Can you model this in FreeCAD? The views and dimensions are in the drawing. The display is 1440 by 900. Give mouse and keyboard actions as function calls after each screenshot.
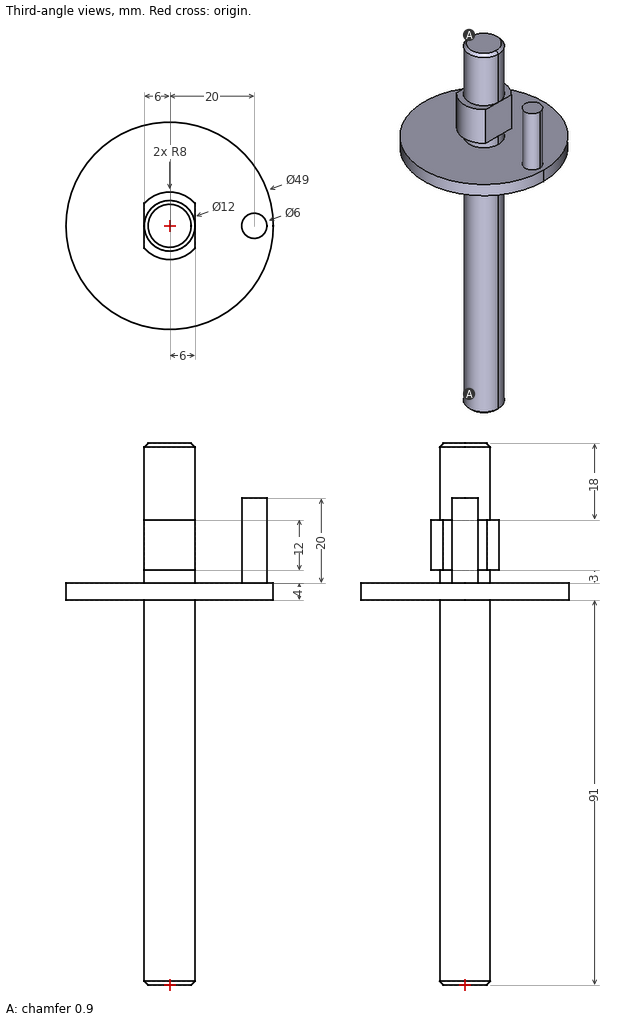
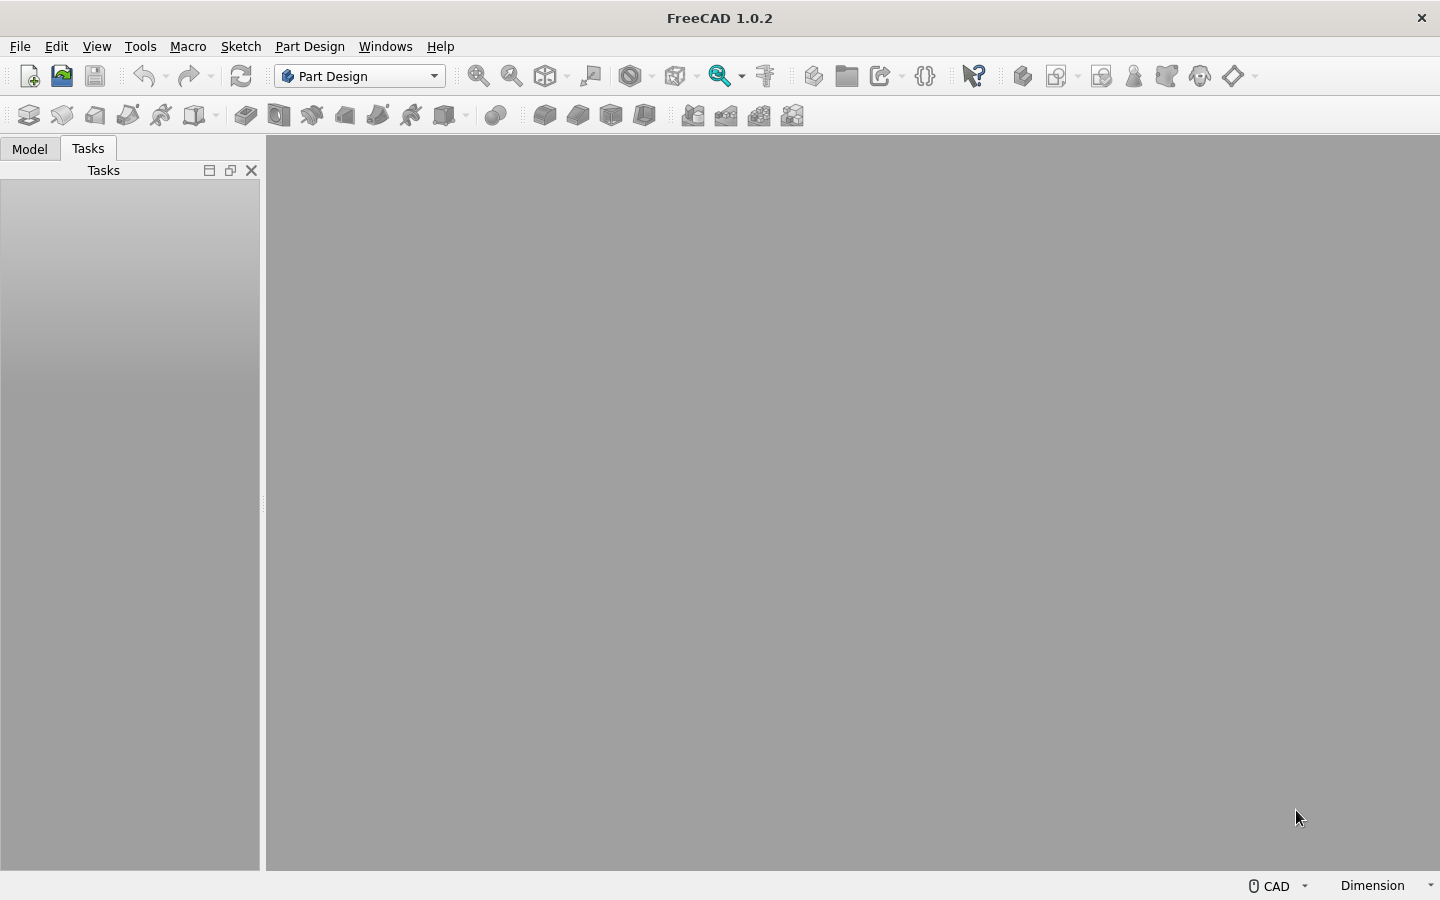
key(ctrl+n)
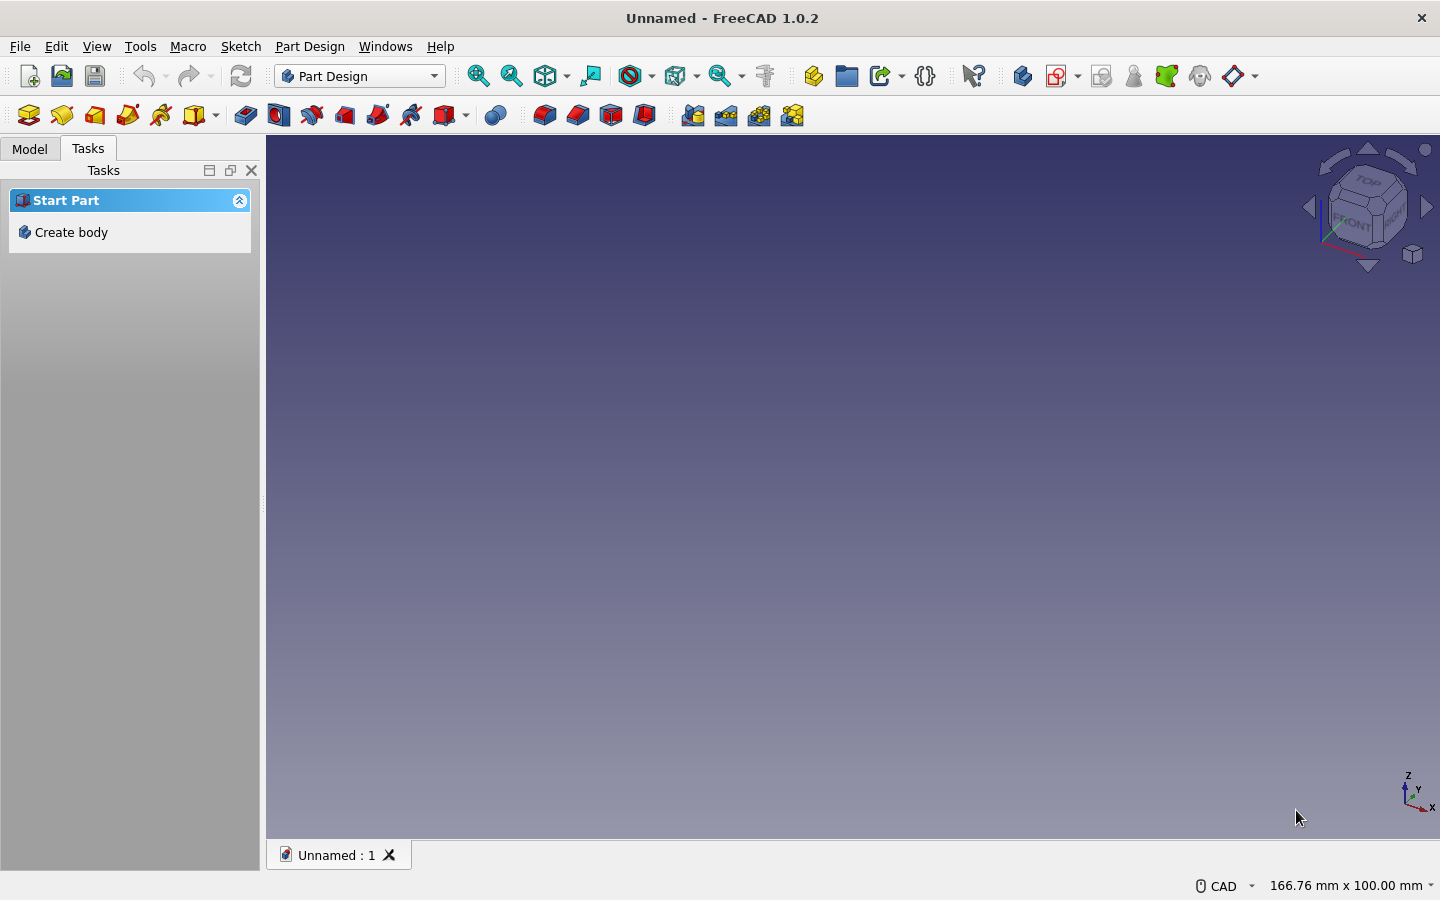
click(1056, 76)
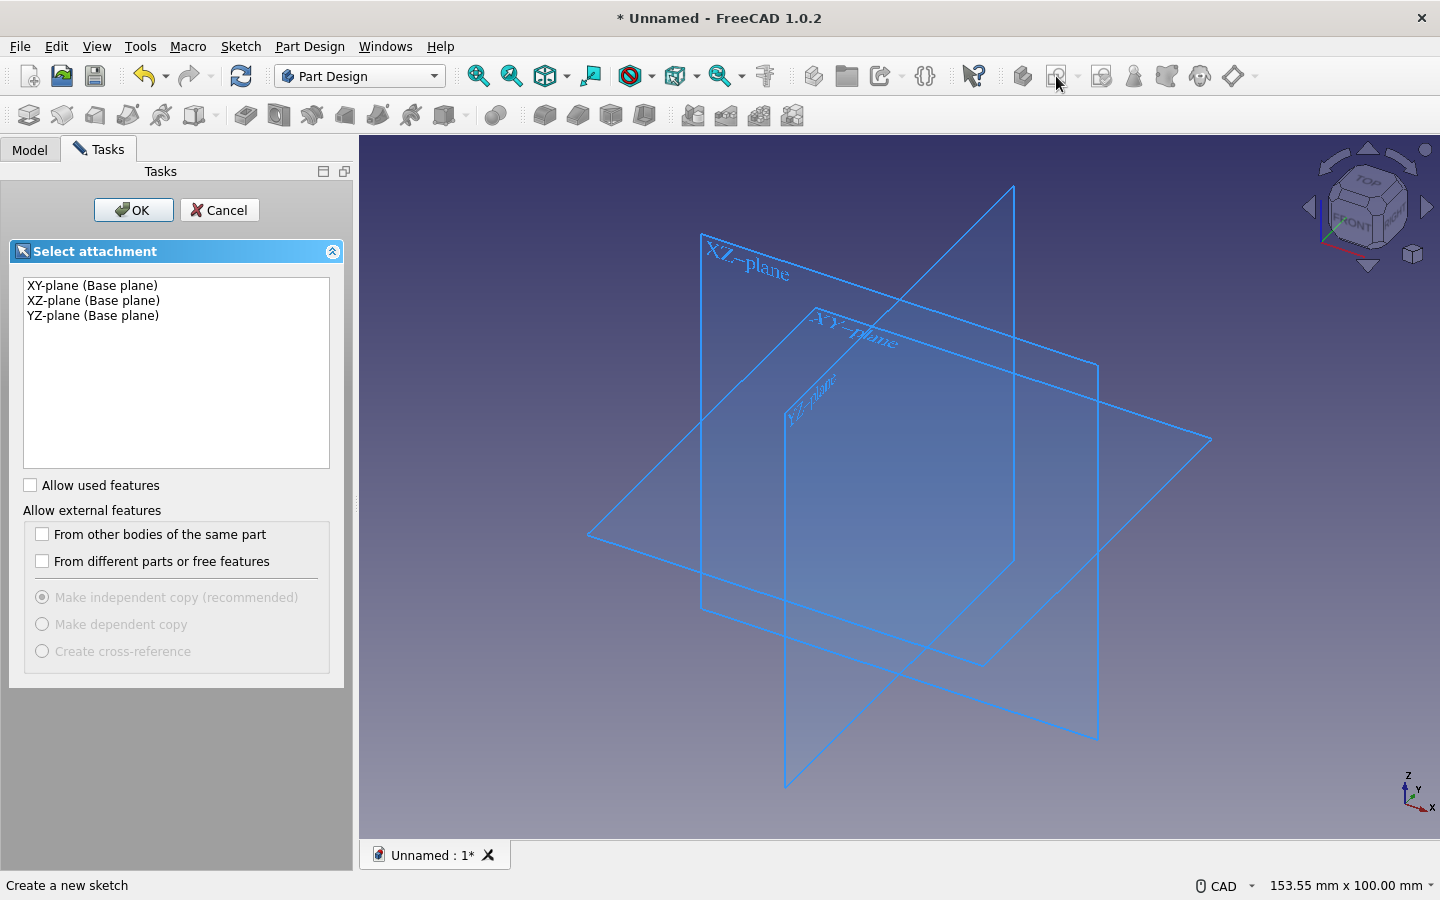
click(84, 286)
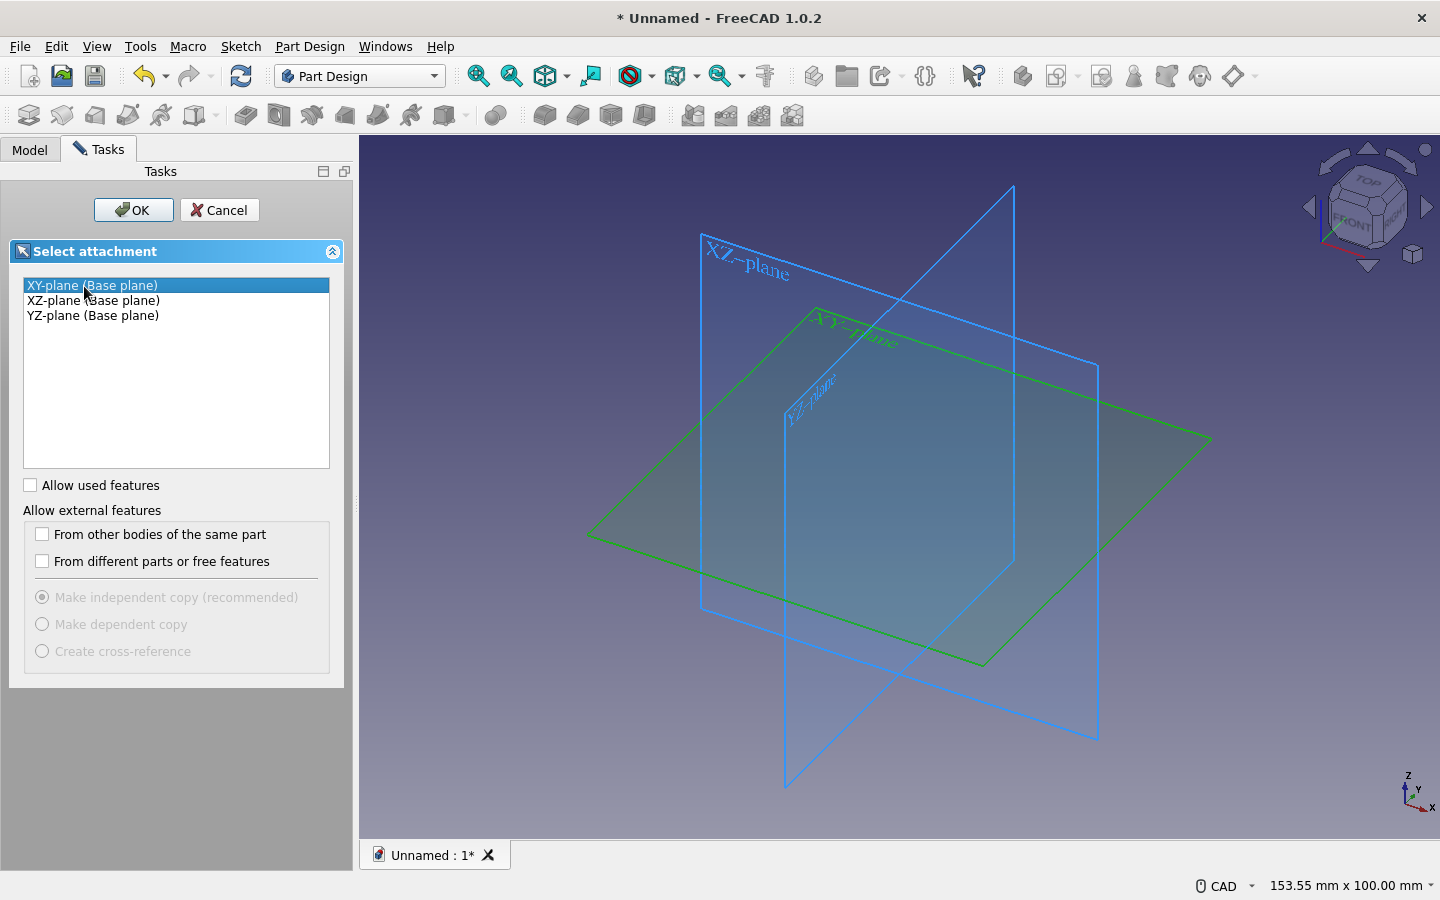
click(134, 210)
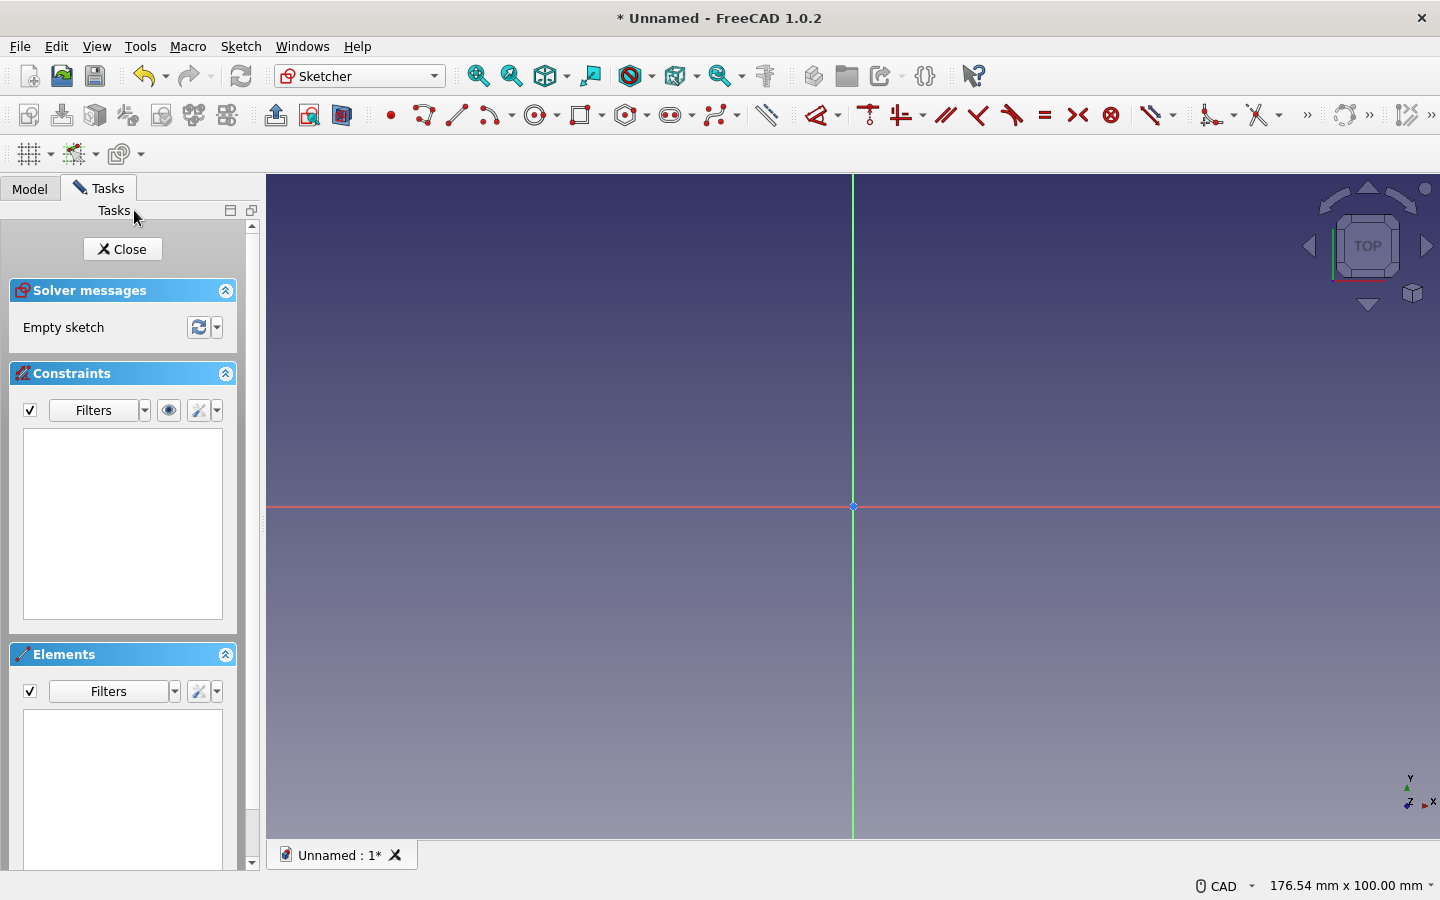
scroll(870, 506, up, 8)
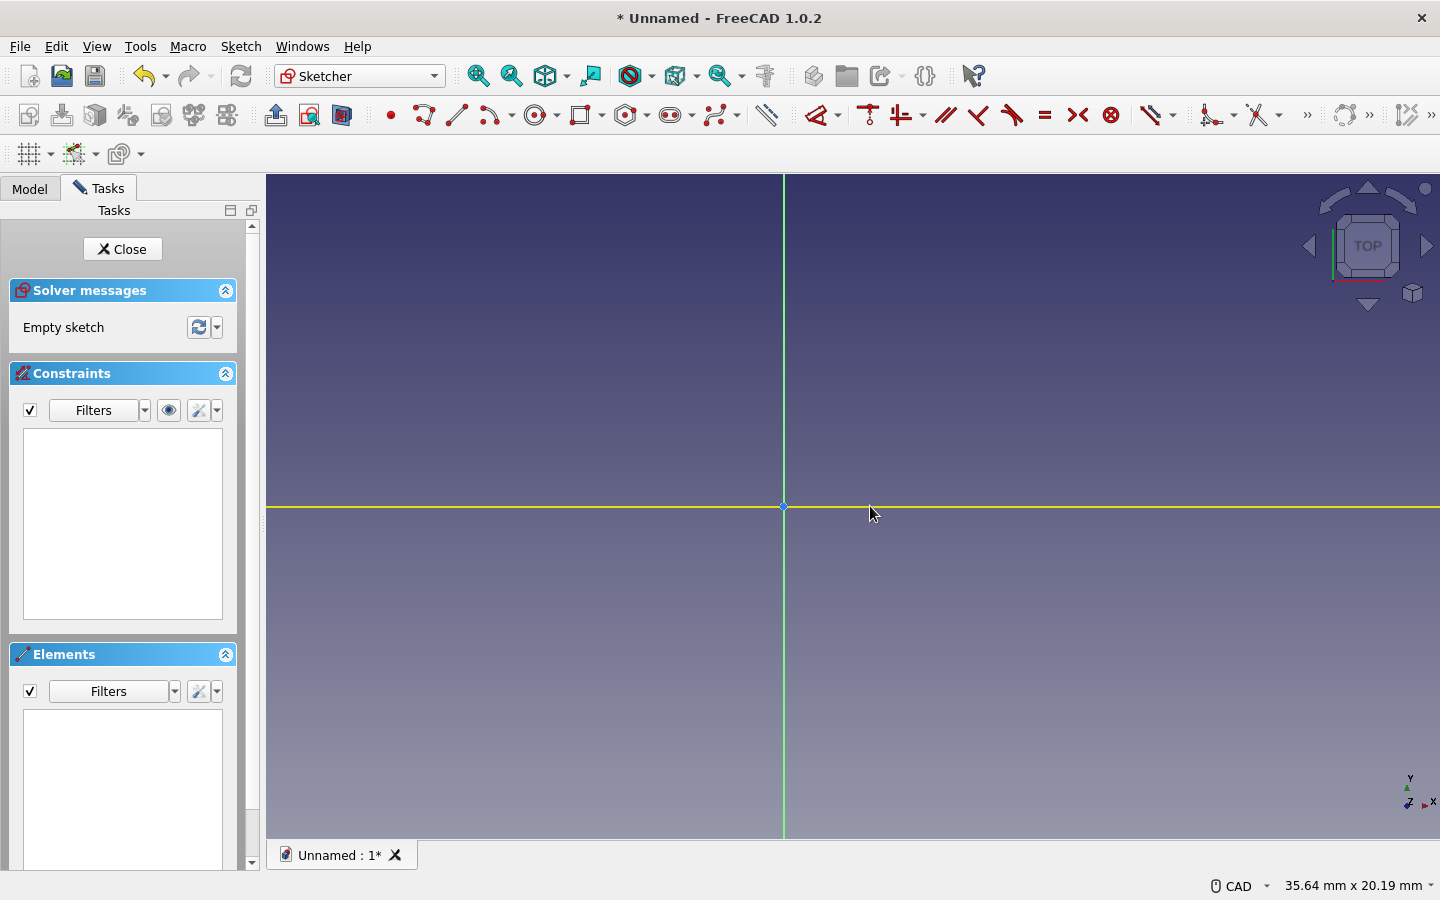
key(g)
key(c)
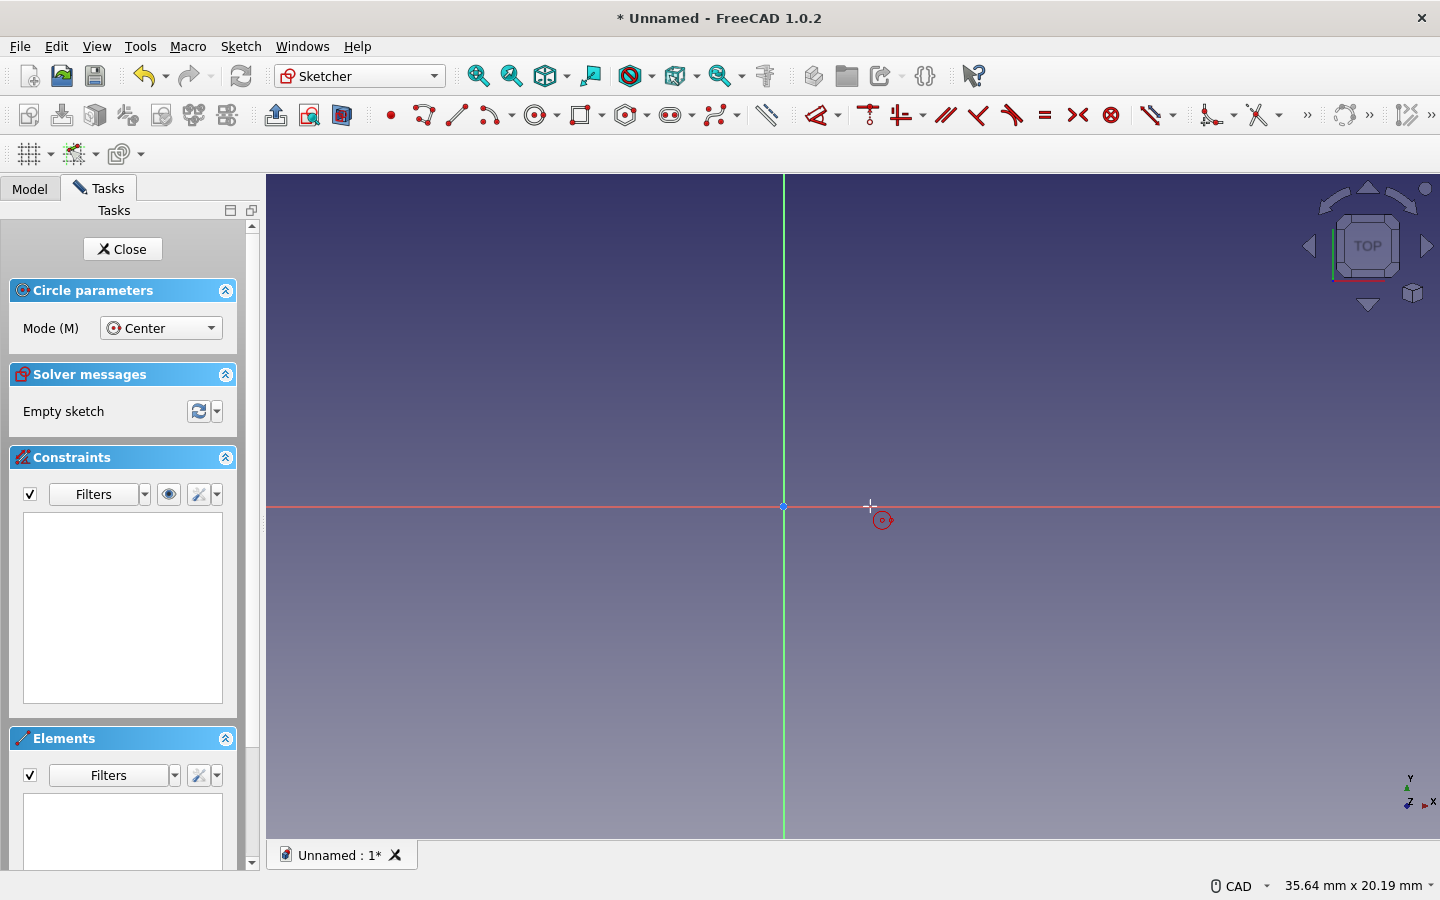
click(784, 506)
click(924, 367)
key(Escape)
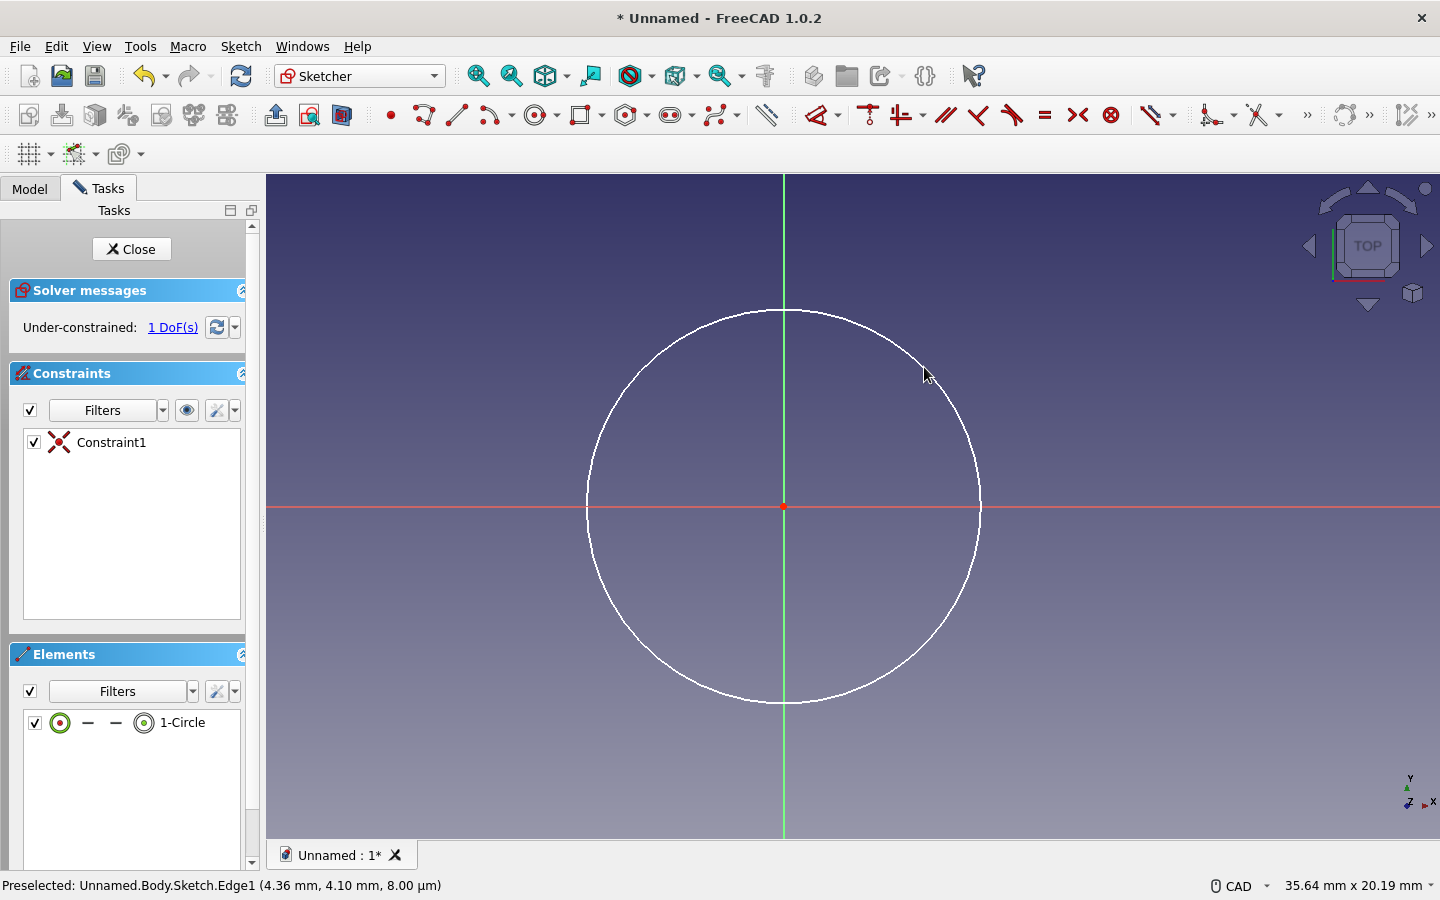
click(923, 367)